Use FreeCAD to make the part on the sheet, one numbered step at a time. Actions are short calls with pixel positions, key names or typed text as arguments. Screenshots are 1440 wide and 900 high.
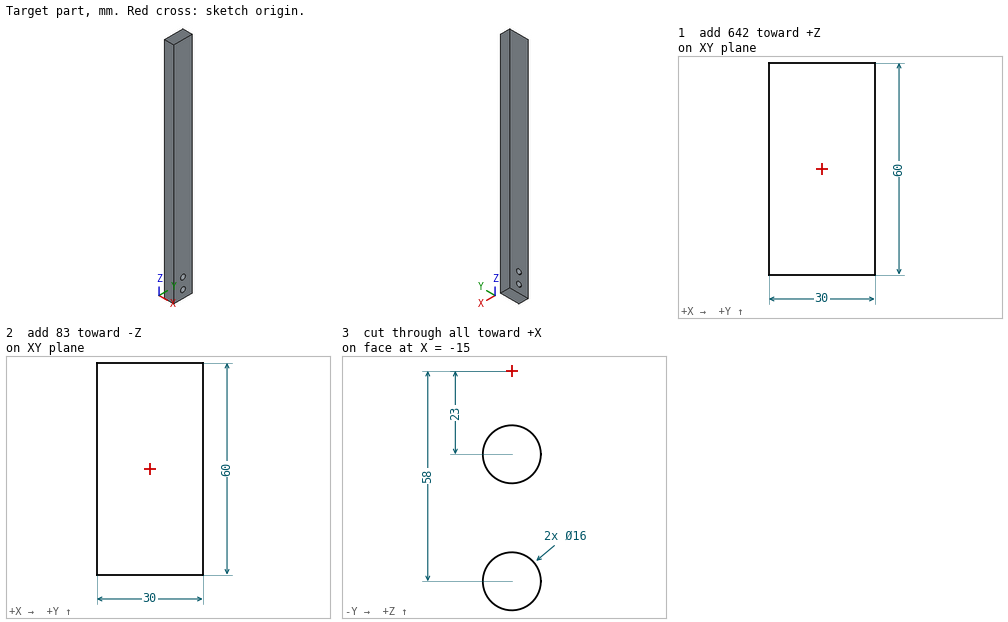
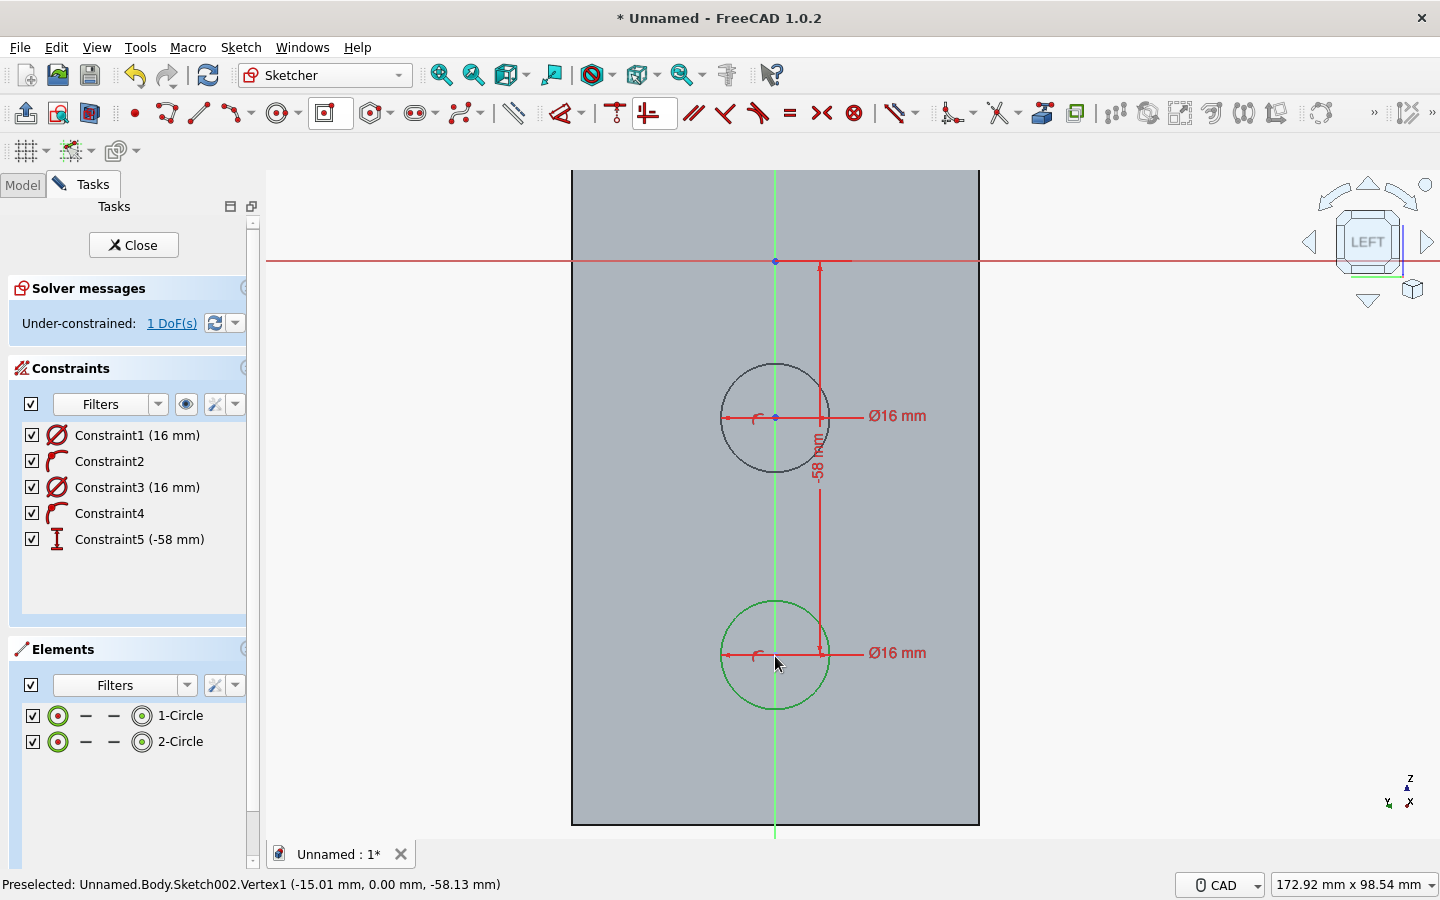
click(775, 418)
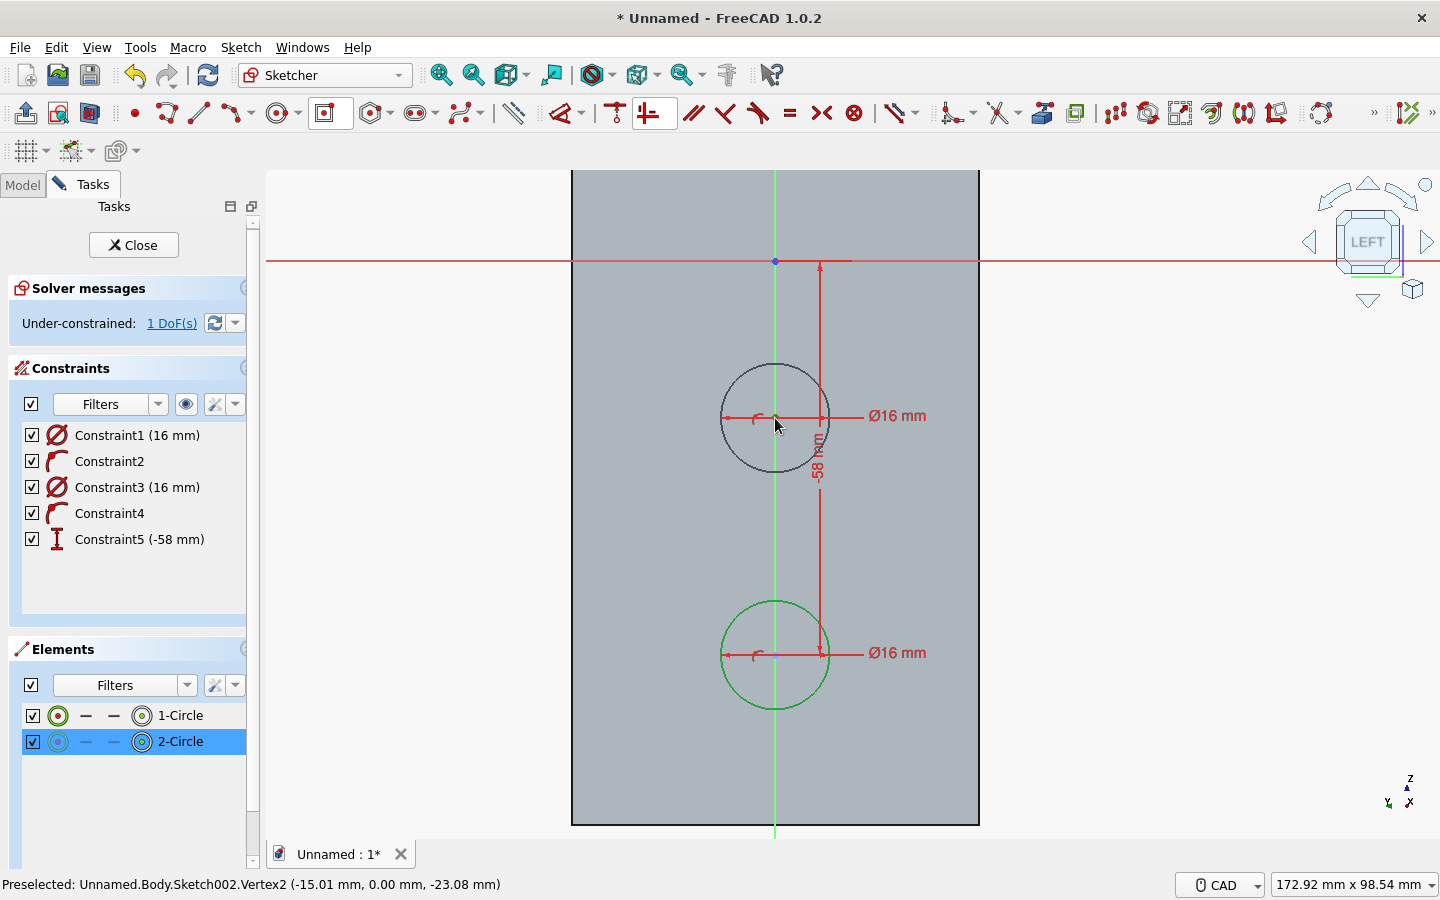
click(584, 114)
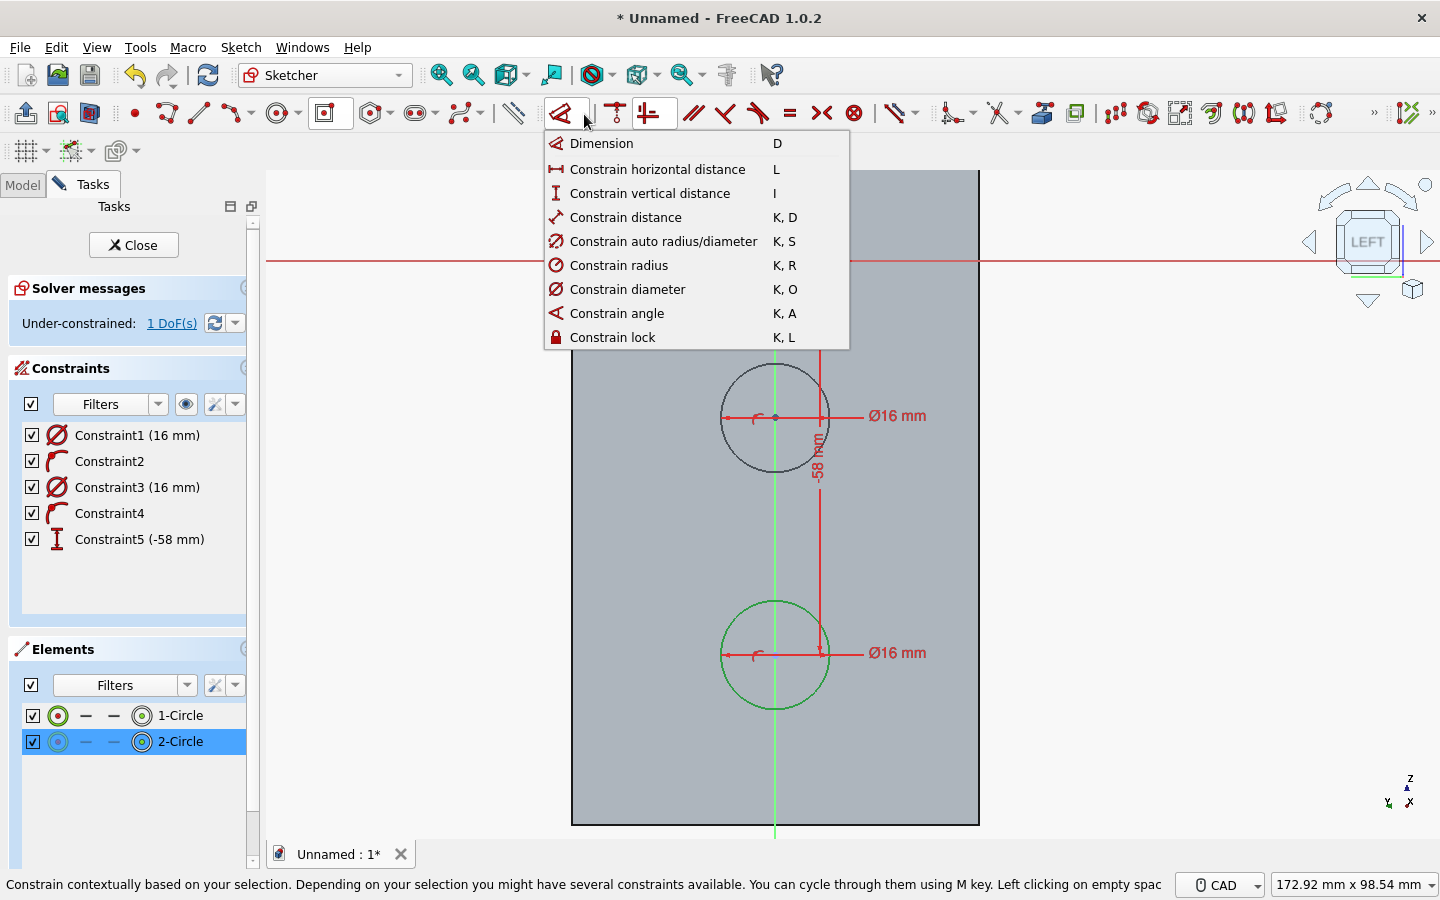
click(697, 193)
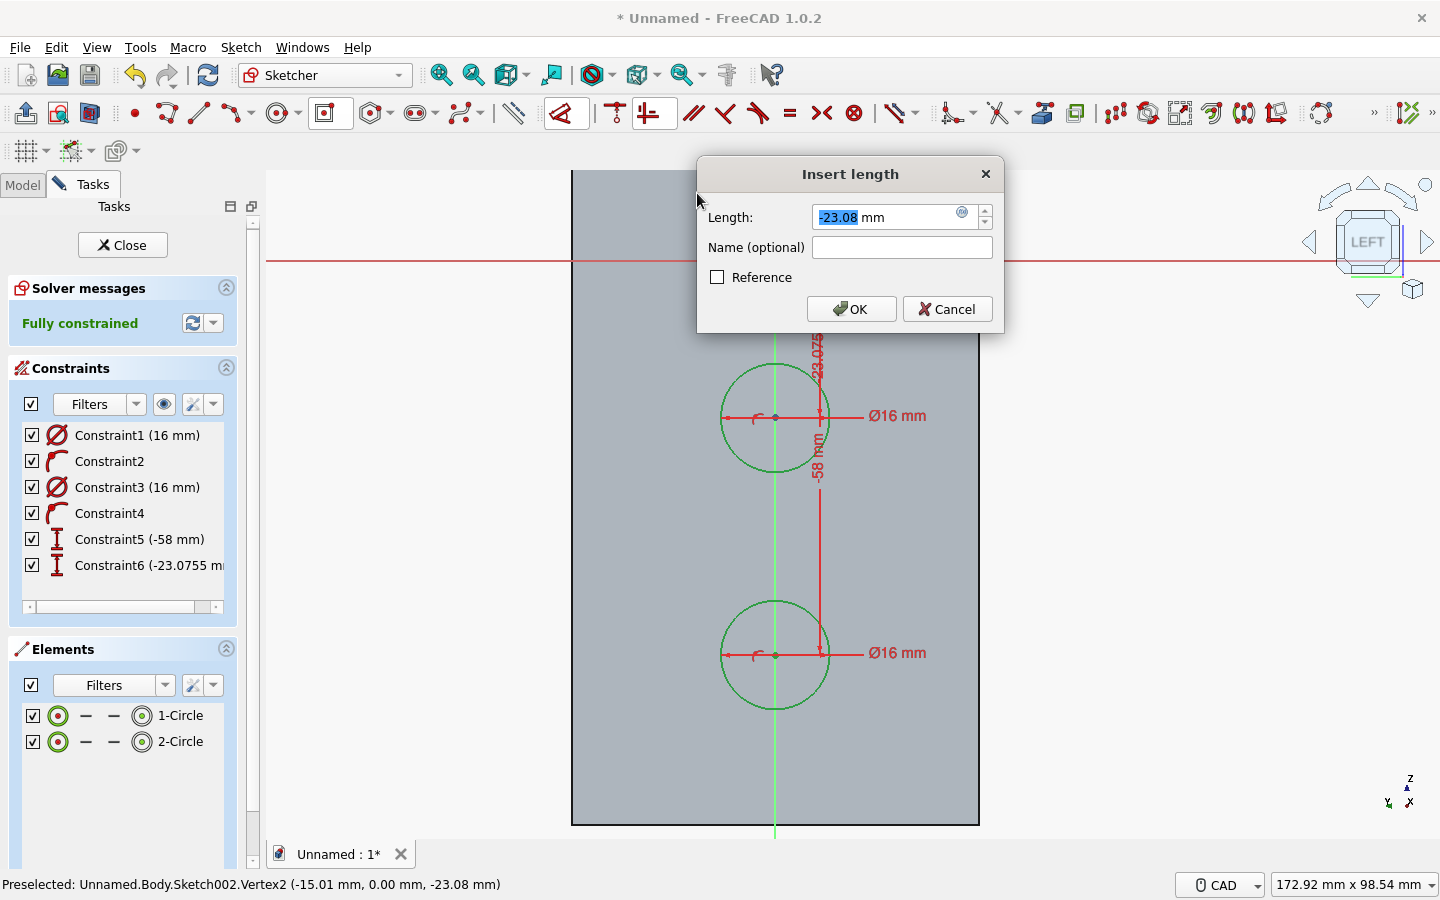
text(-23)
key(Return)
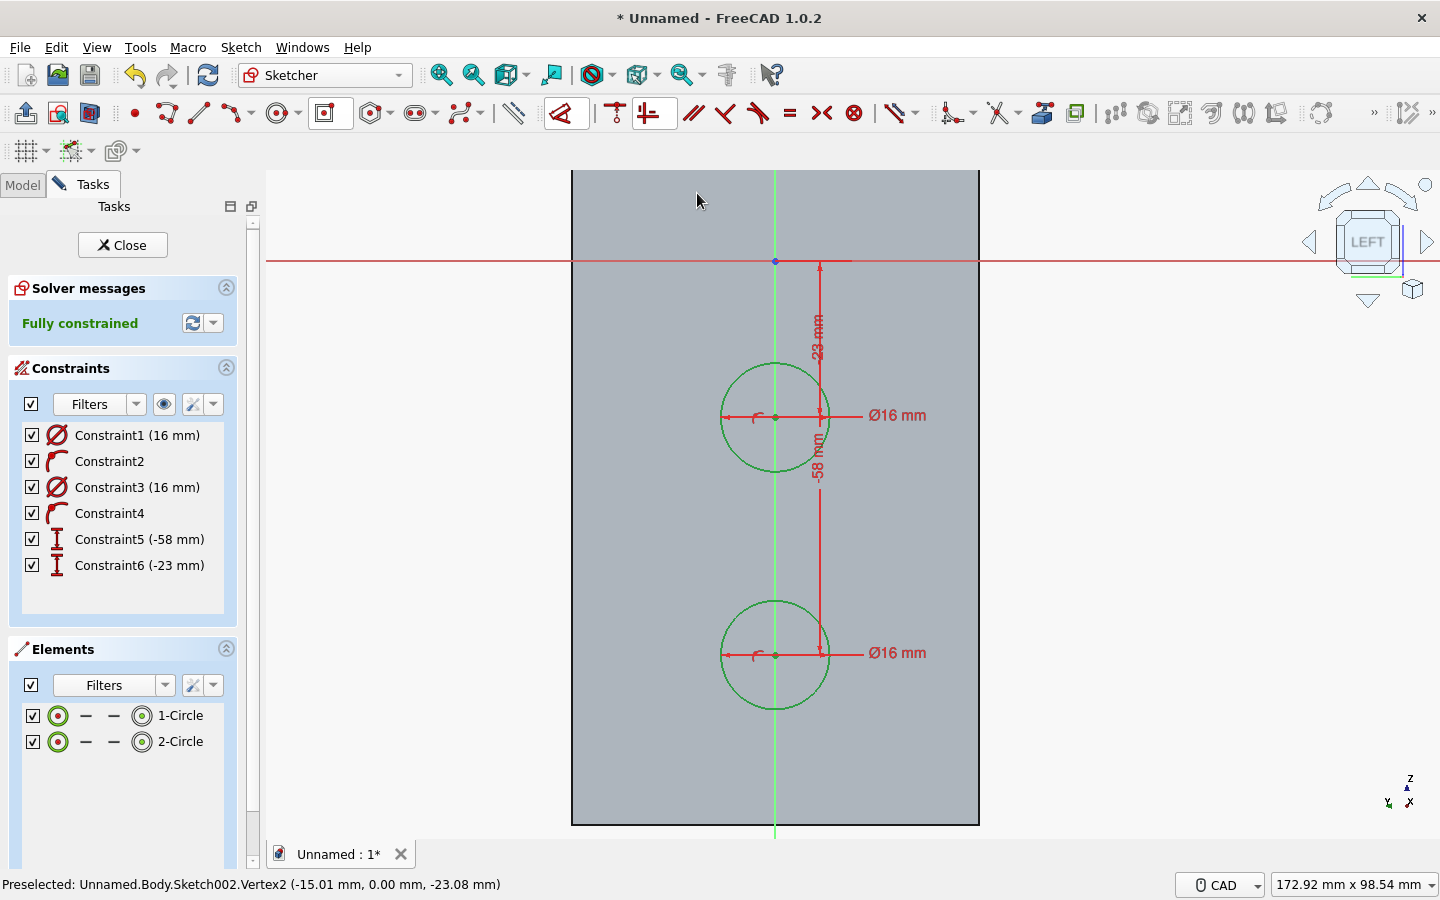
click(123, 245)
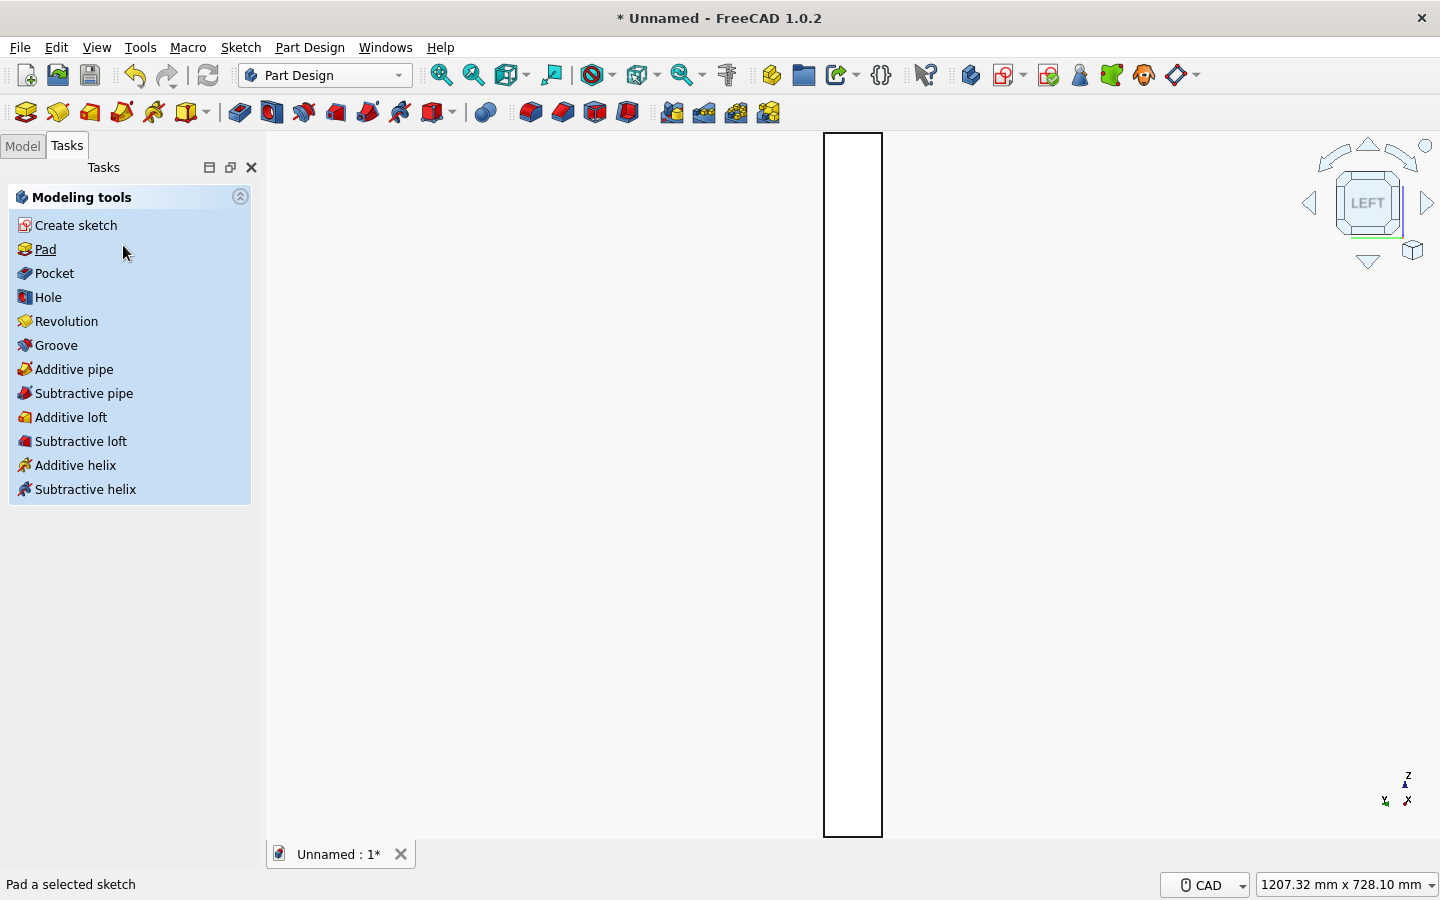
click(240, 112)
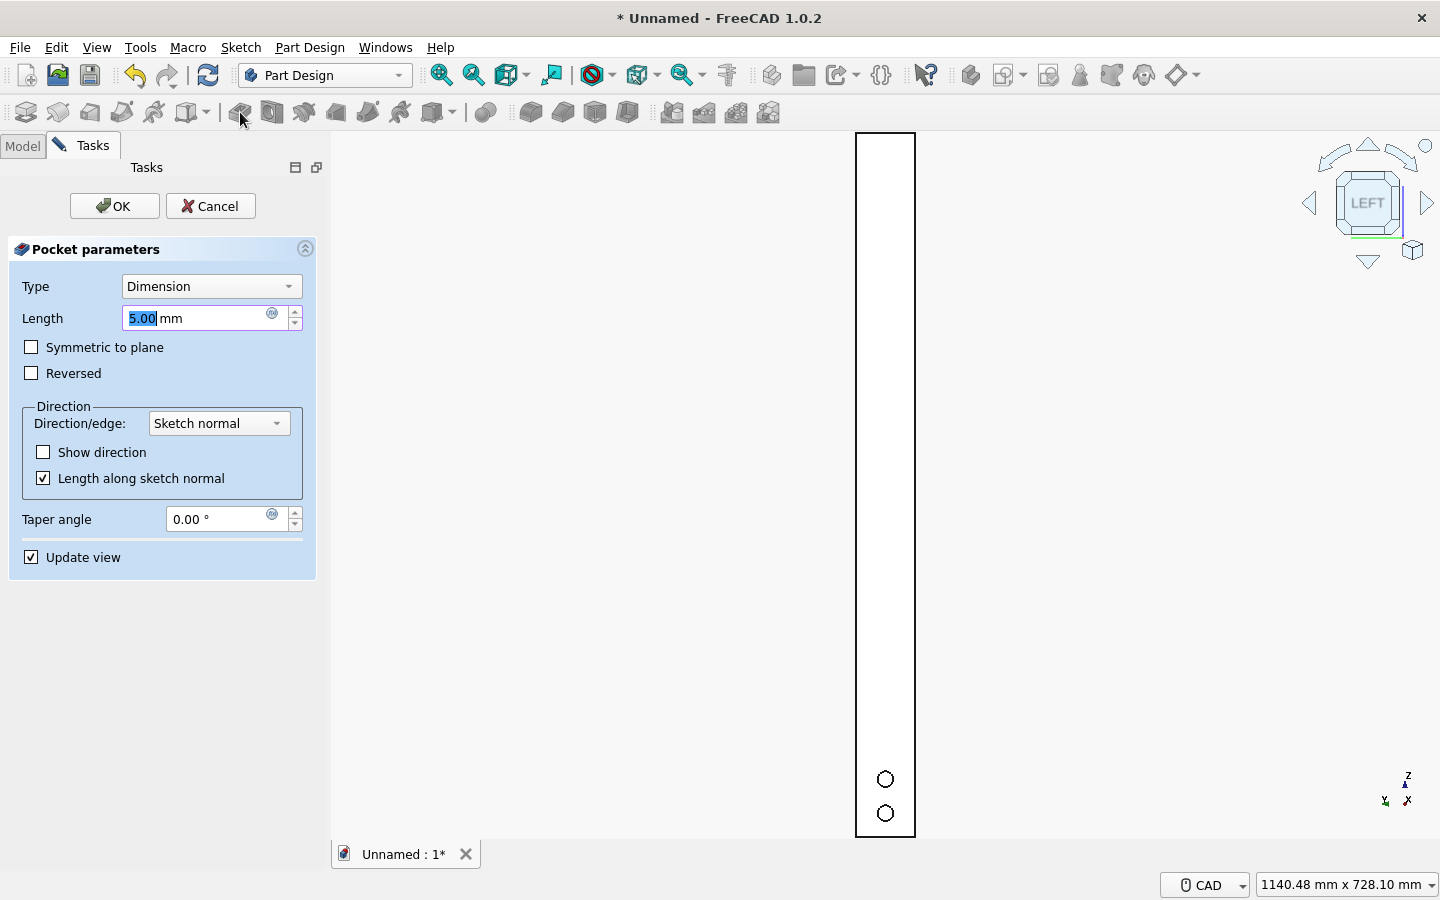
click(212, 286)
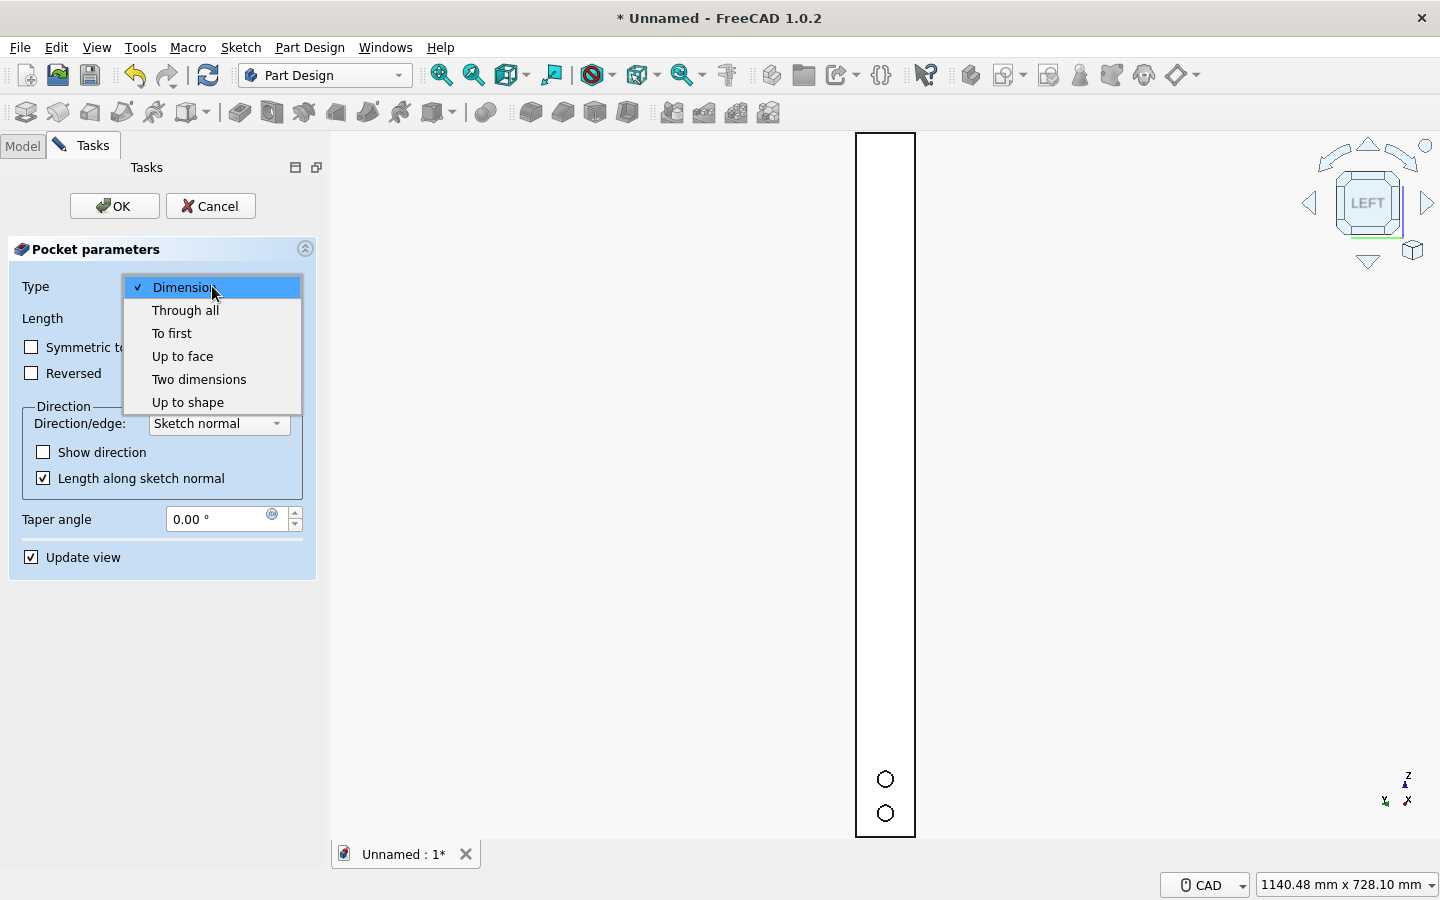
click(212, 310)